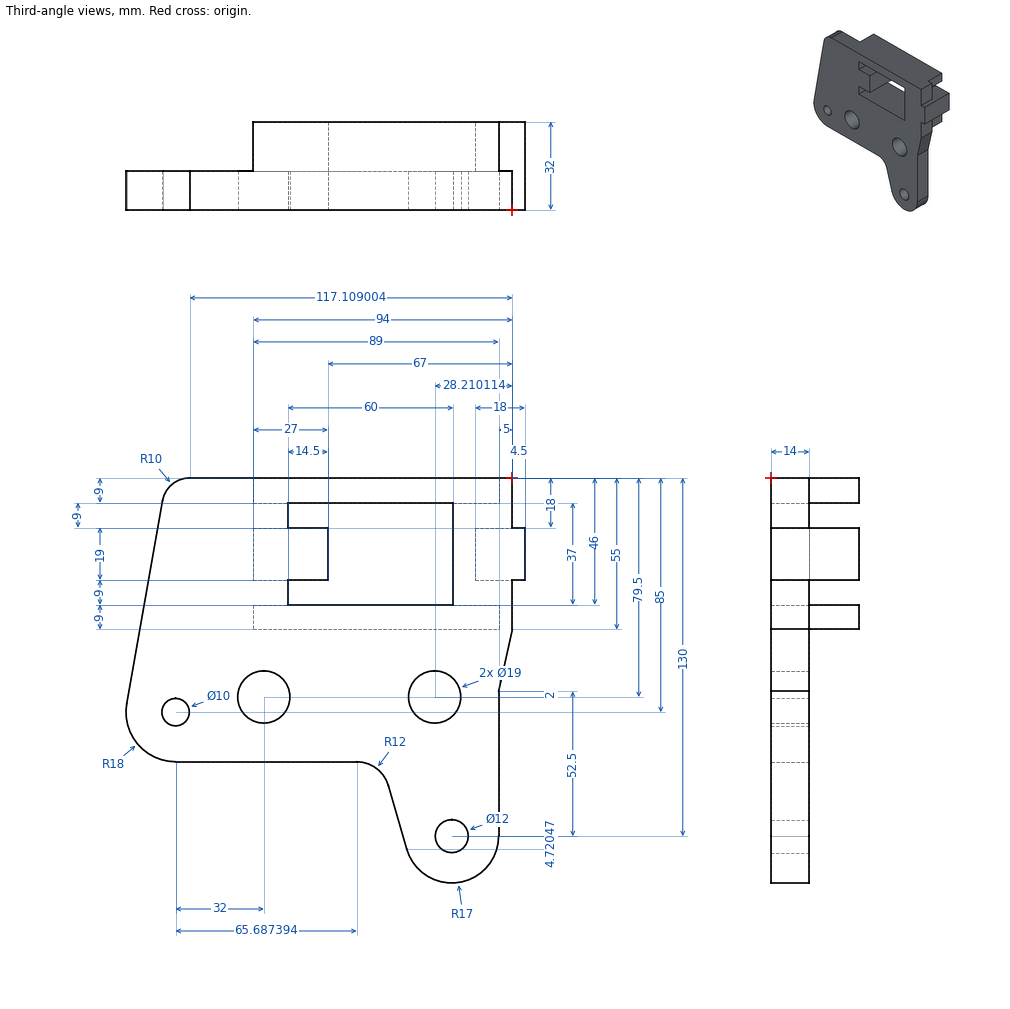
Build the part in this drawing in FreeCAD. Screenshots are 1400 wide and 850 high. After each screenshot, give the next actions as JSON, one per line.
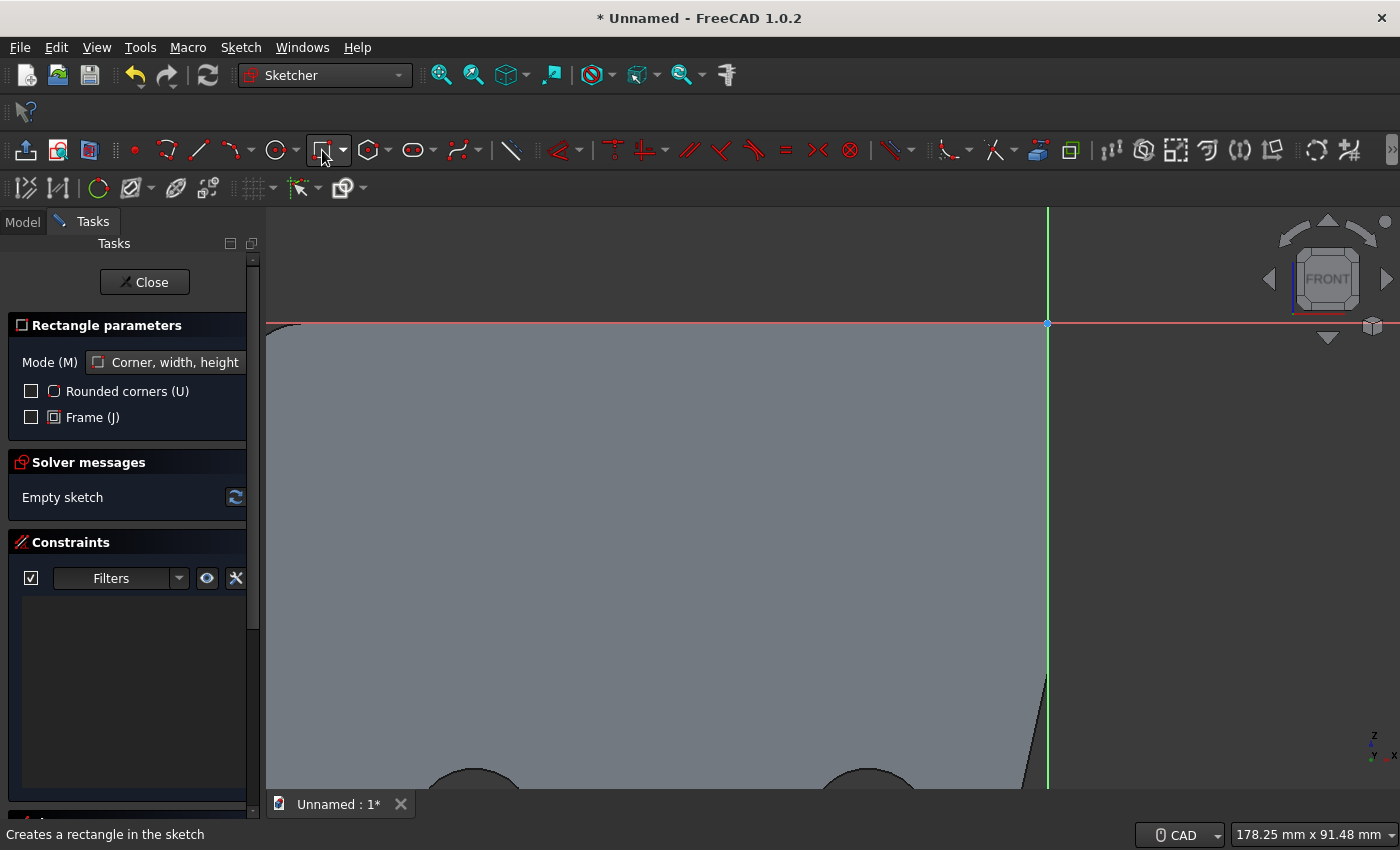
{"action": "left_click", "coordinate": [450, 323]}
{"action": "left_click", "coordinate": [1016, 381]}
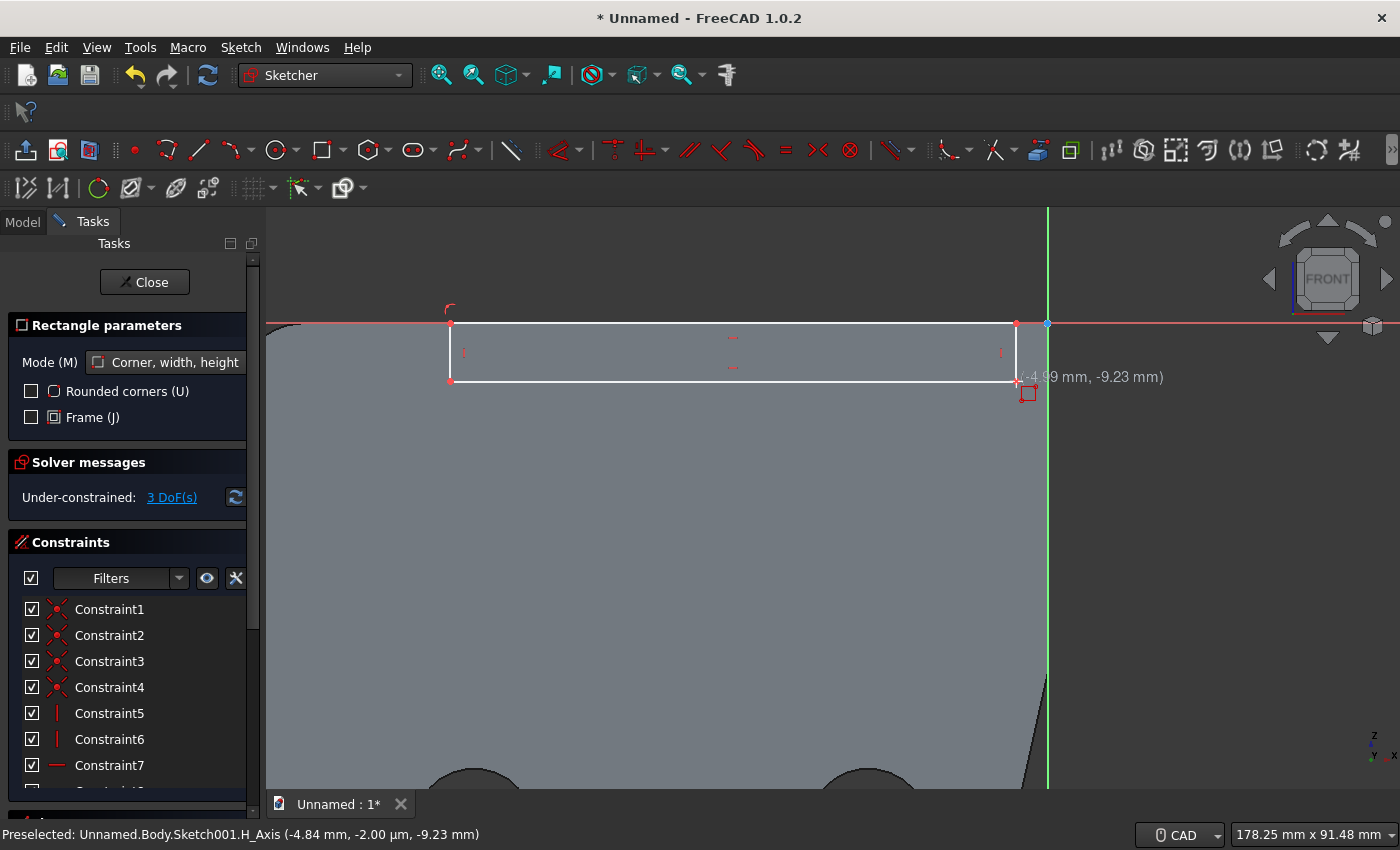
{"action": "left_click", "coordinate": [450, 438]}
{"action": "left_click", "coordinate": [622, 559]}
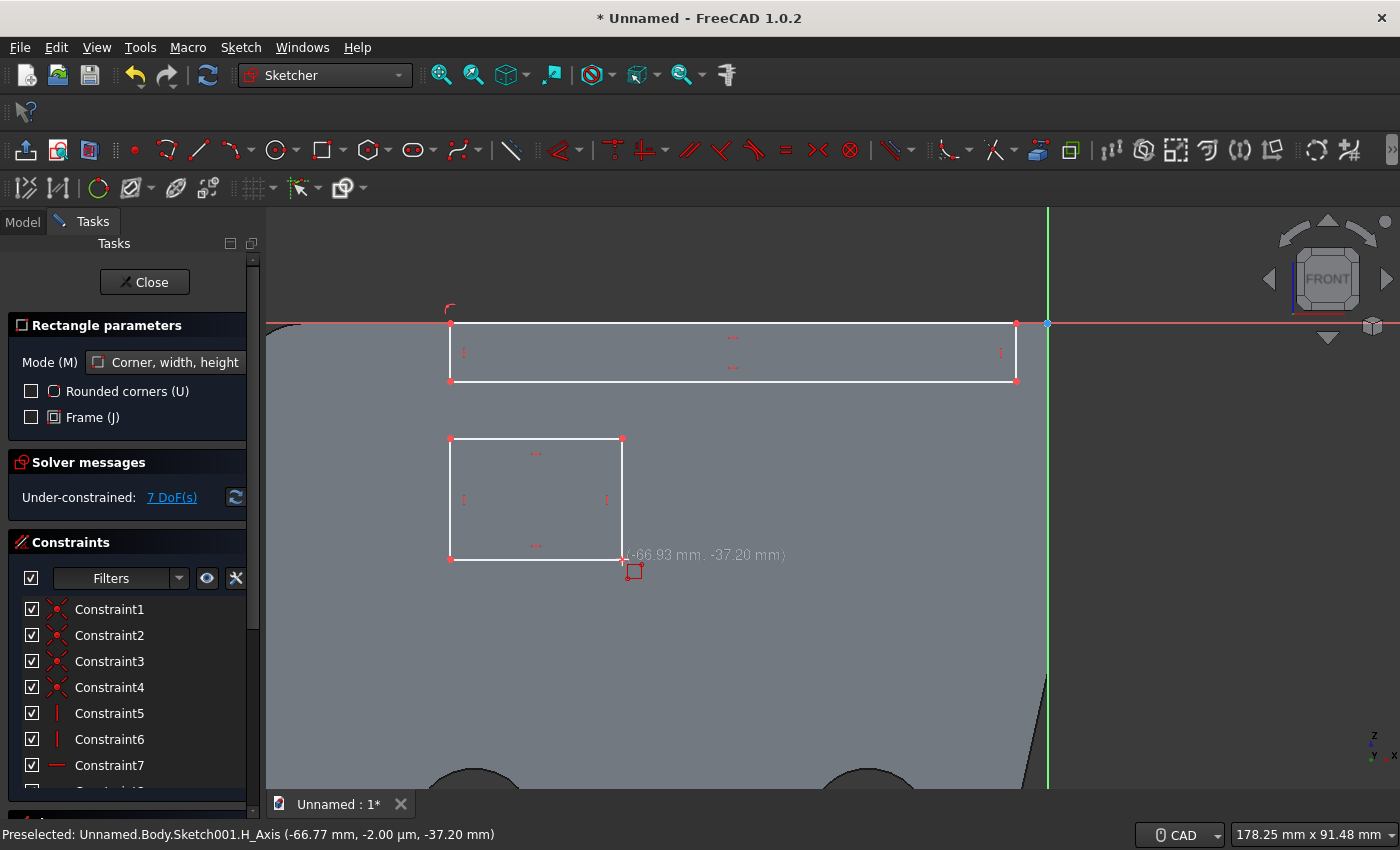
{"action": "left_click", "coordinate": [450, 616]}
{"action": "left_click", "coordinate": [1016, 673]}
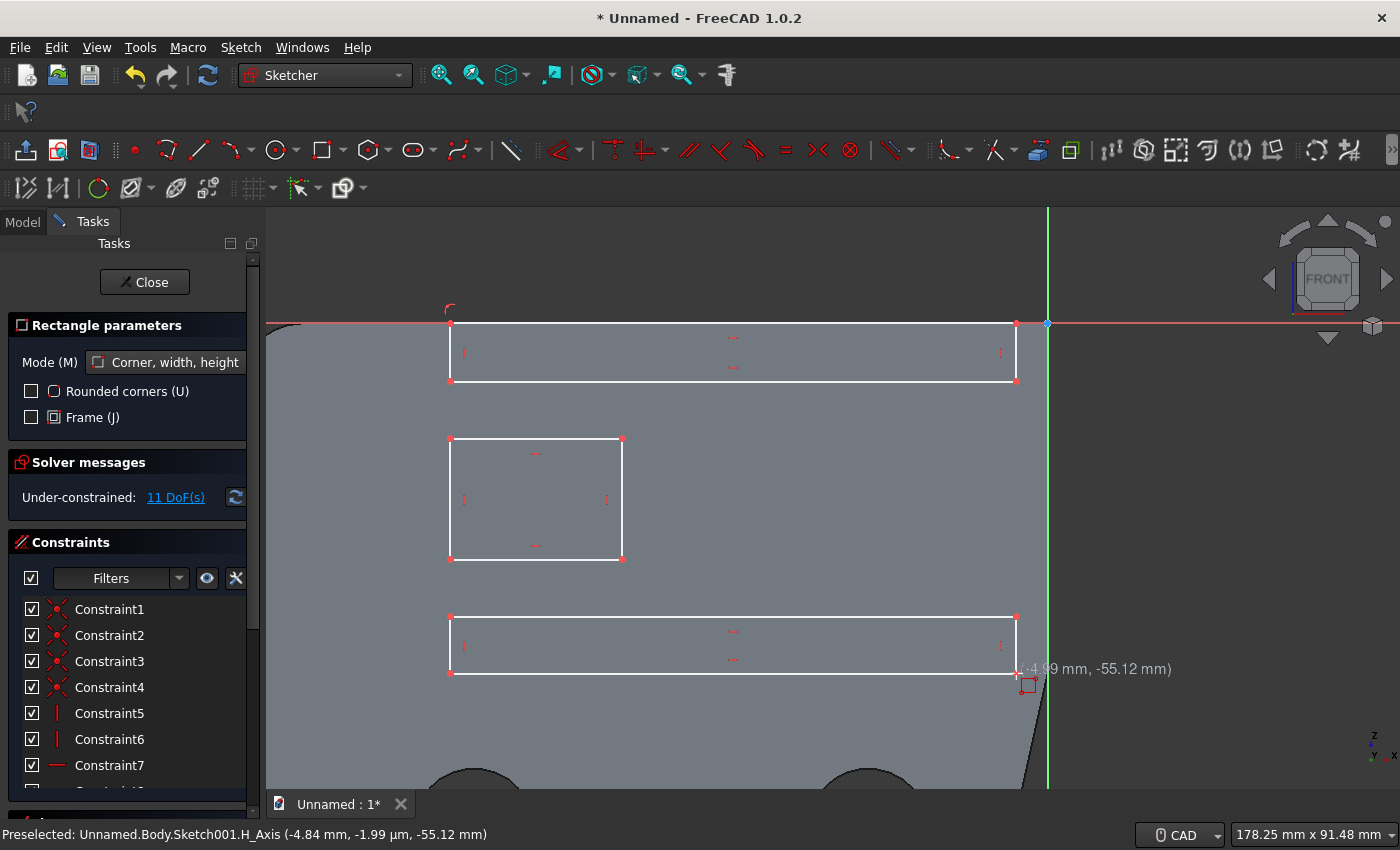
{"action": "left_click", "coordinate": [962, 438]}
{"action": "left_click", "coordinate": [1076, 559]}
{"action": "key", "text": "Escape"}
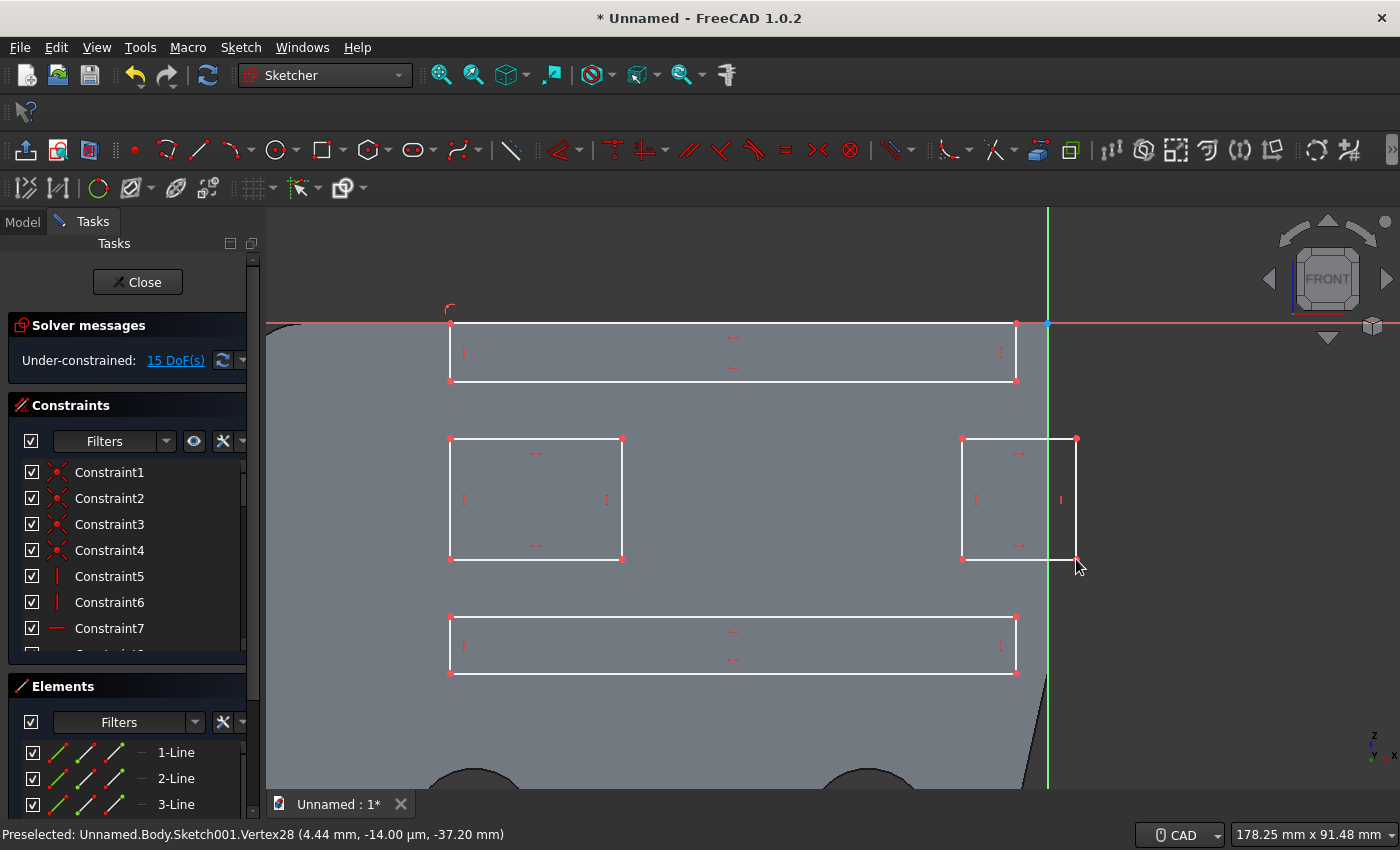
{"action": "left_click", "coordinate": [558, 150]}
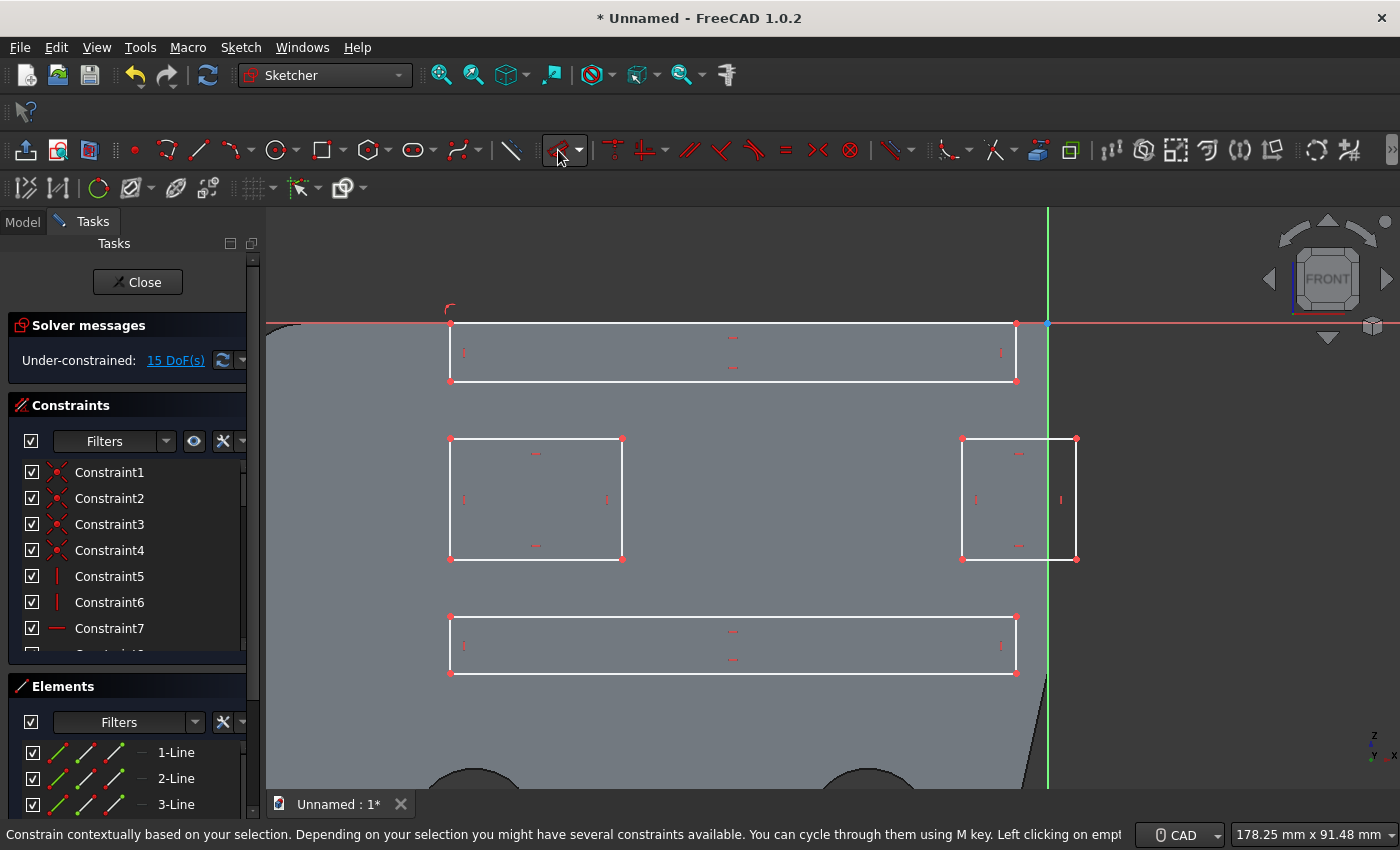
{"action": "left_click", "coordinate": [450, 341]}
{"action": "left_click", "coordinate": [416, 353]}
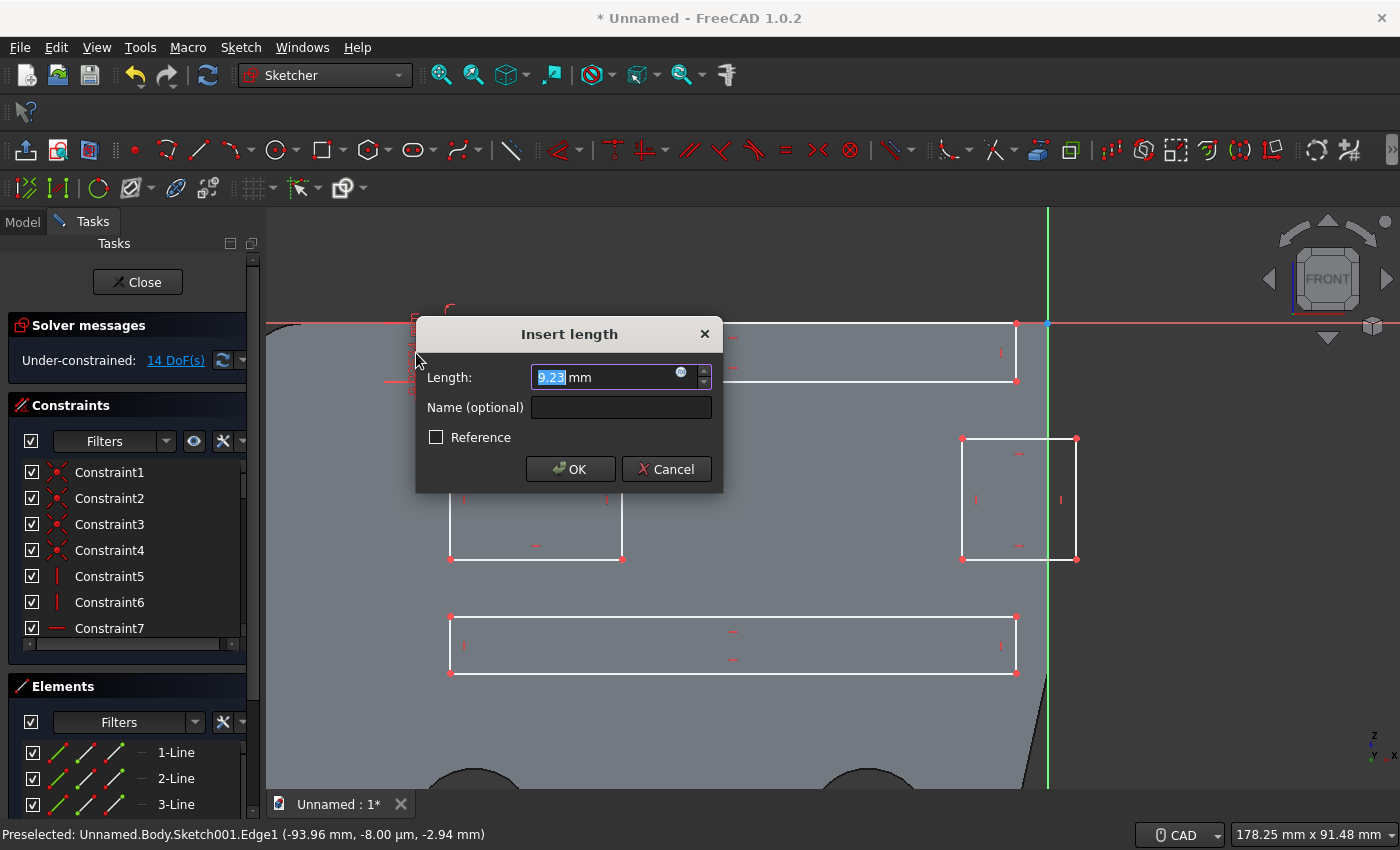
{"action": "type", "text": "9"}
{"action": "key", "text": "Return"}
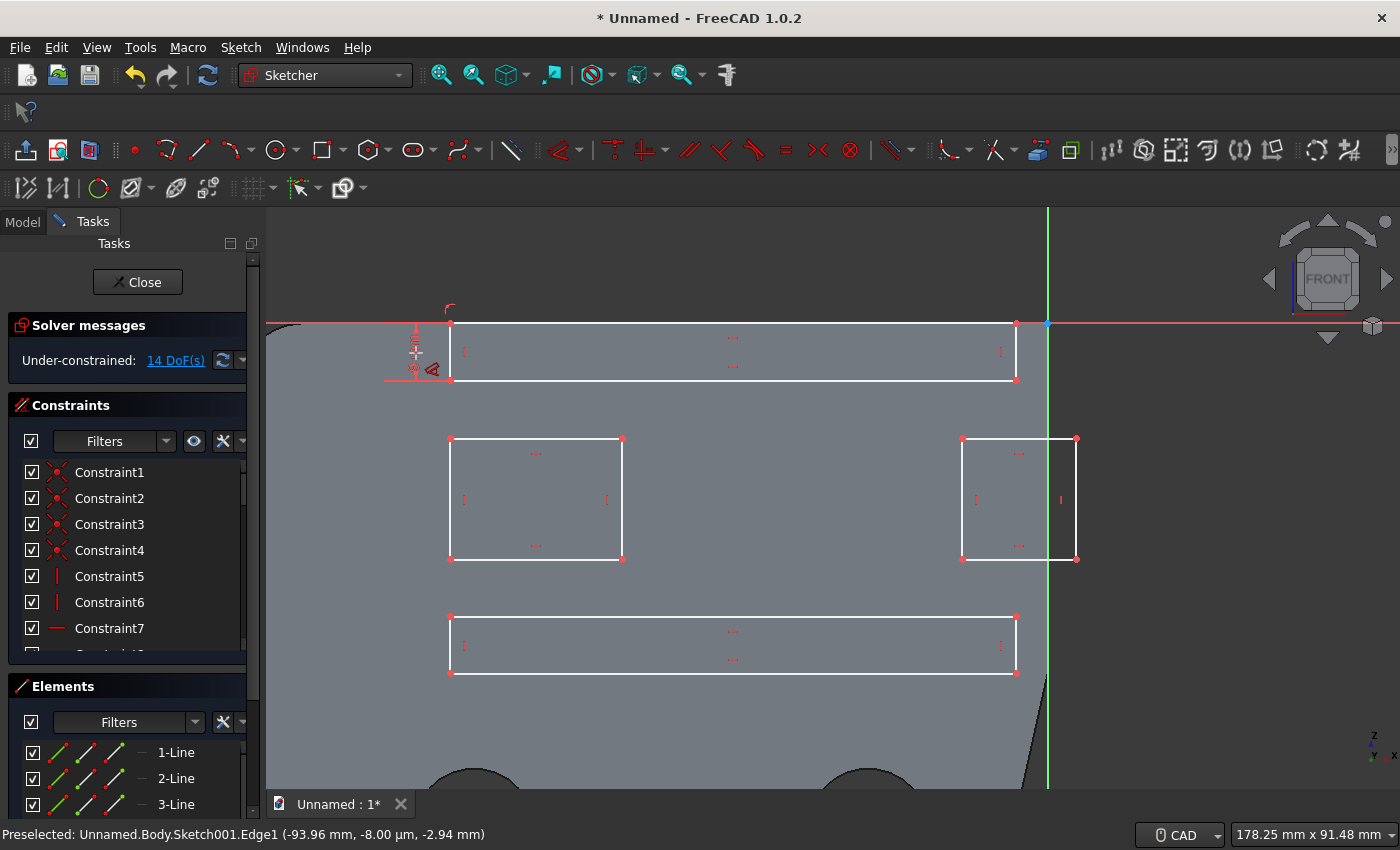
{"action": "left_click", "coordinate": [450, 634]}
{"action": "left_click", "coordinate": [416, 645]}